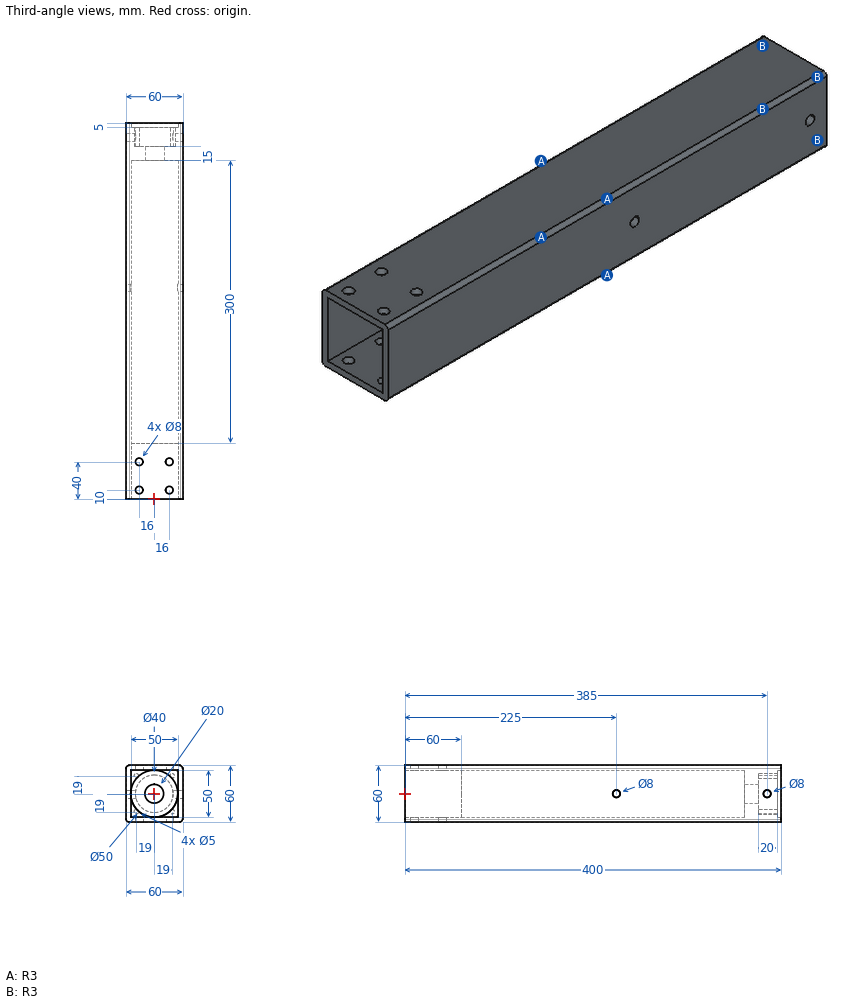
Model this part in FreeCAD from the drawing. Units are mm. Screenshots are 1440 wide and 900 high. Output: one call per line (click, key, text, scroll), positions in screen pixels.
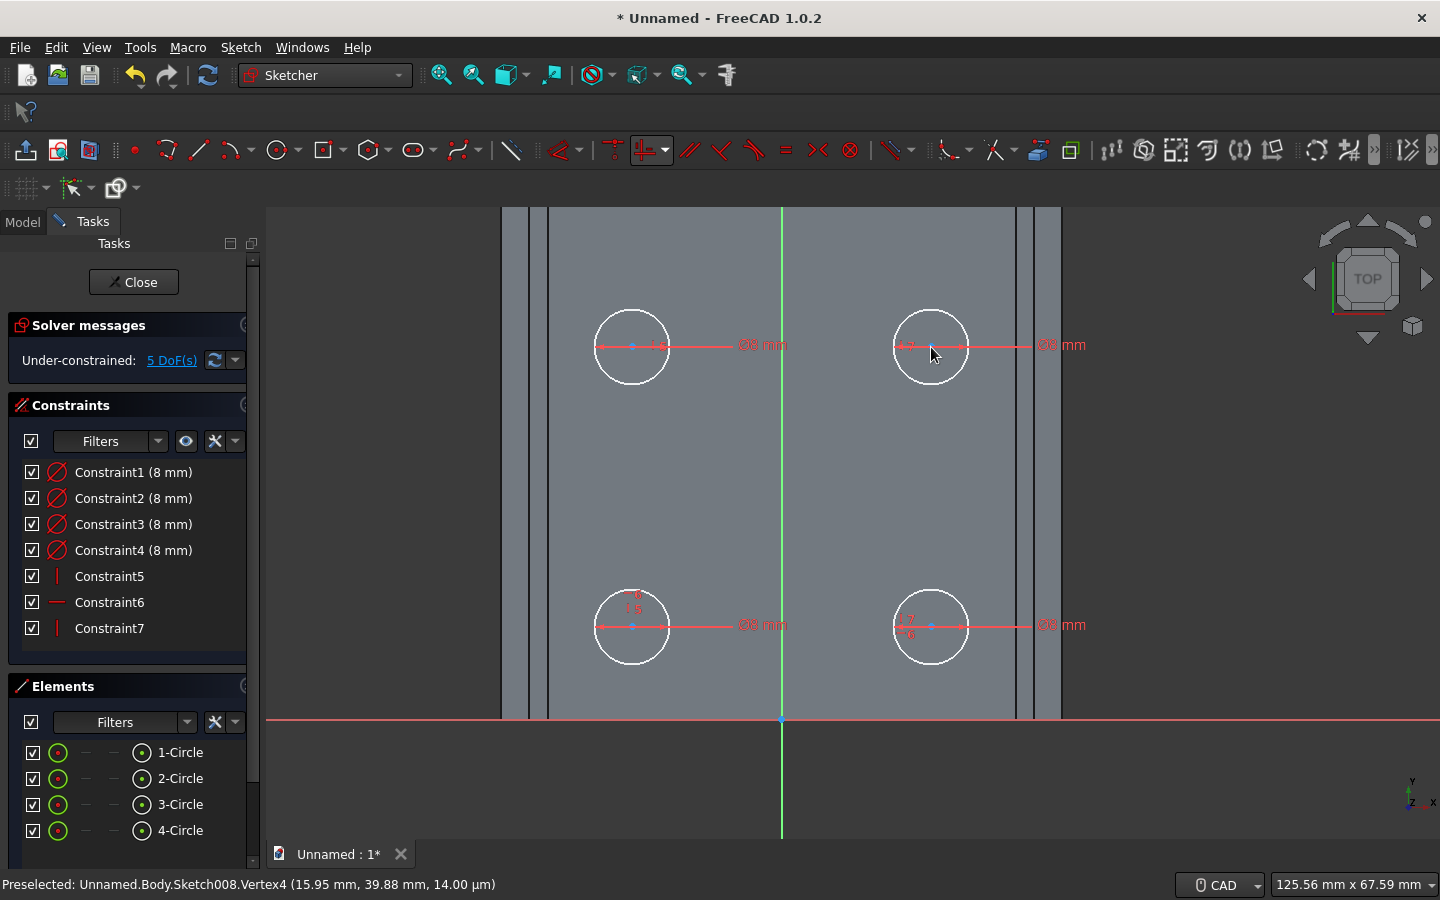
click(632, 347)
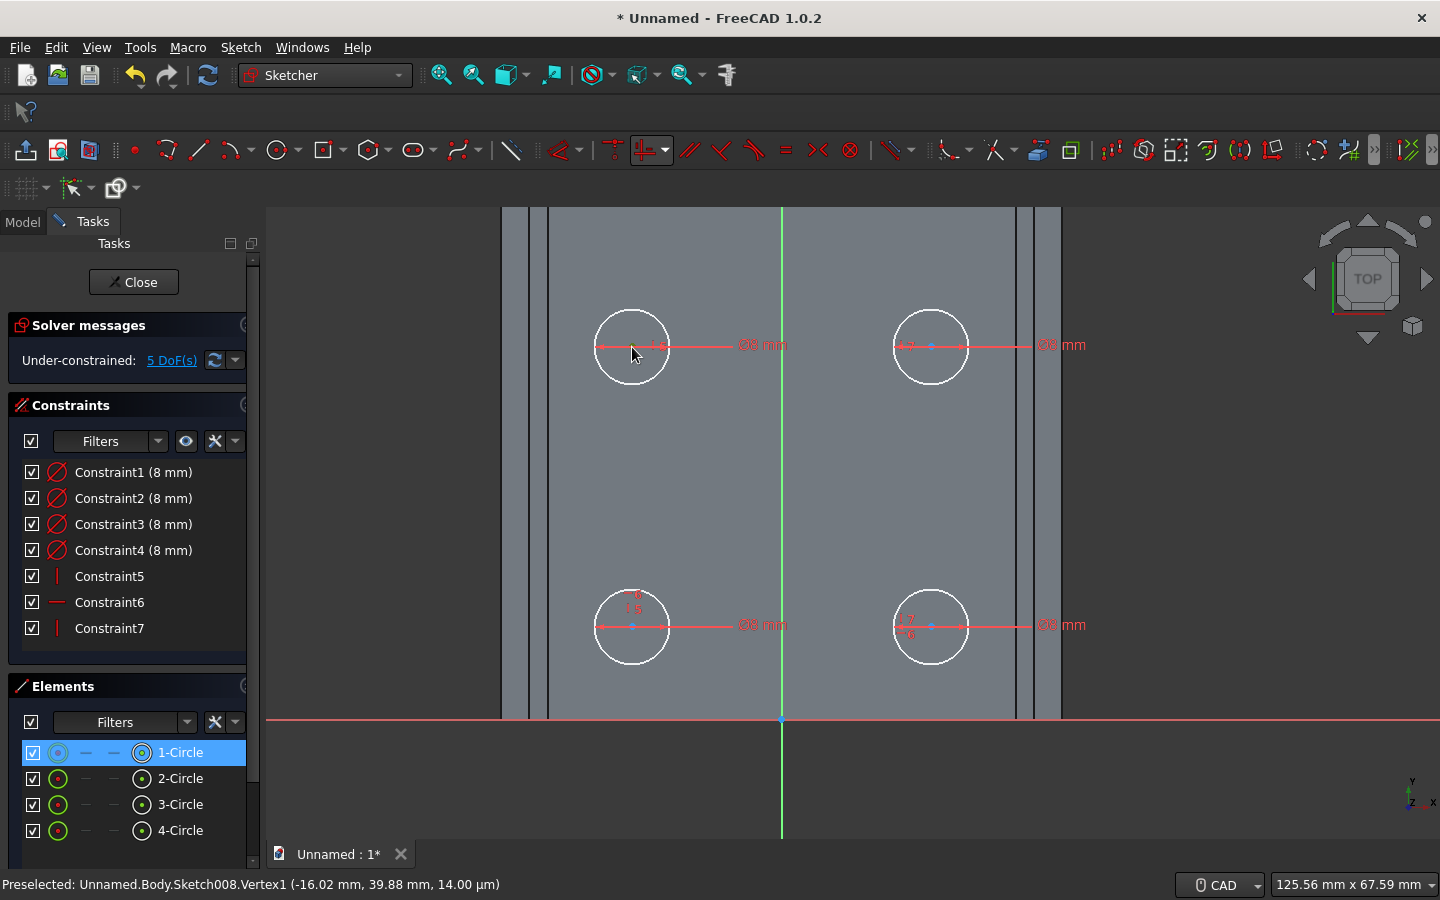
click(931, 347)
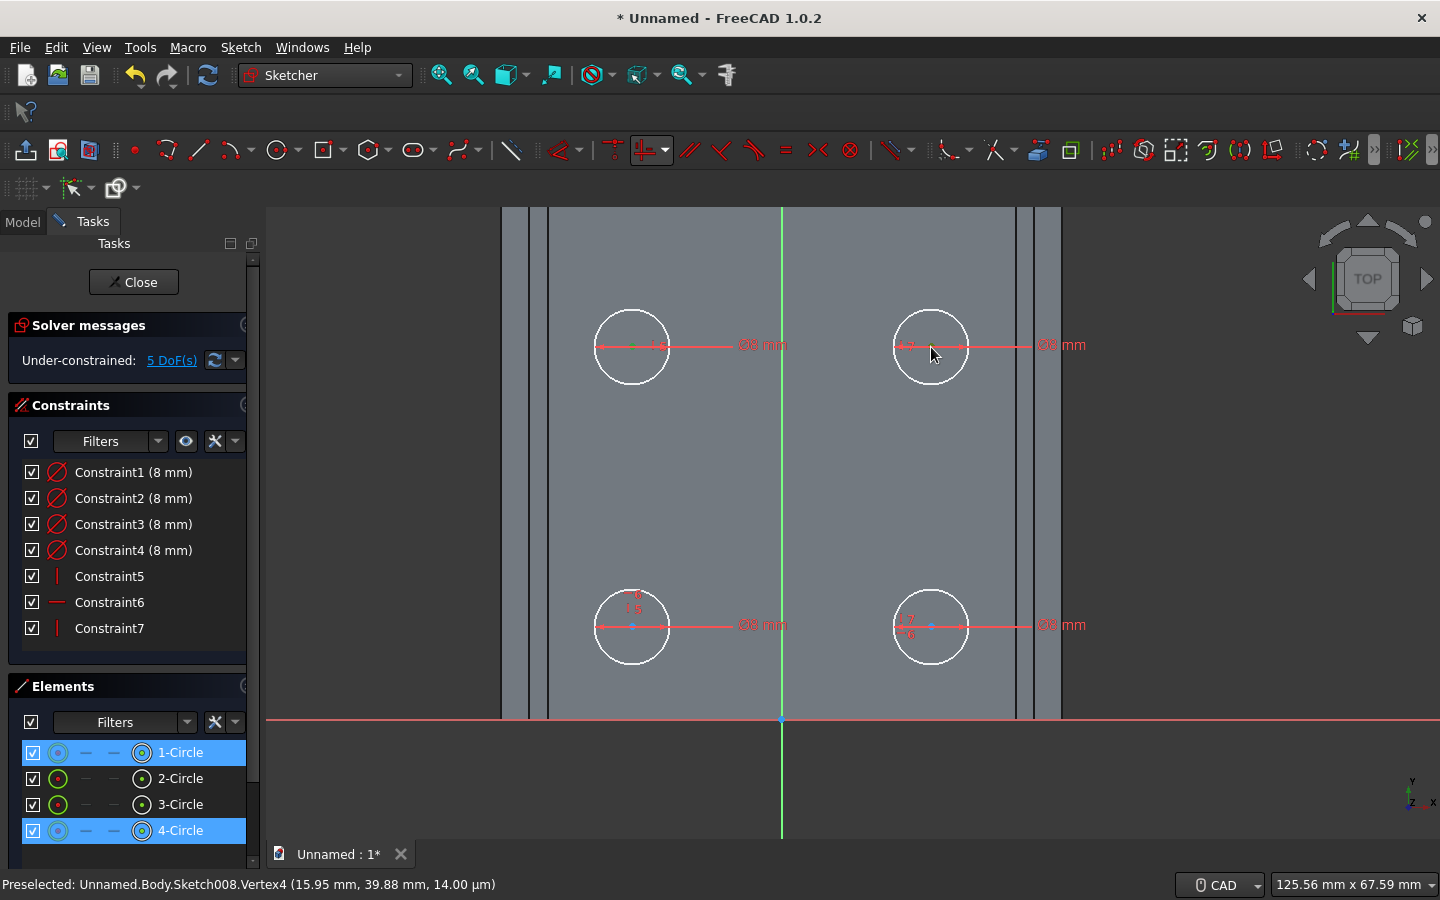
click(668, 150)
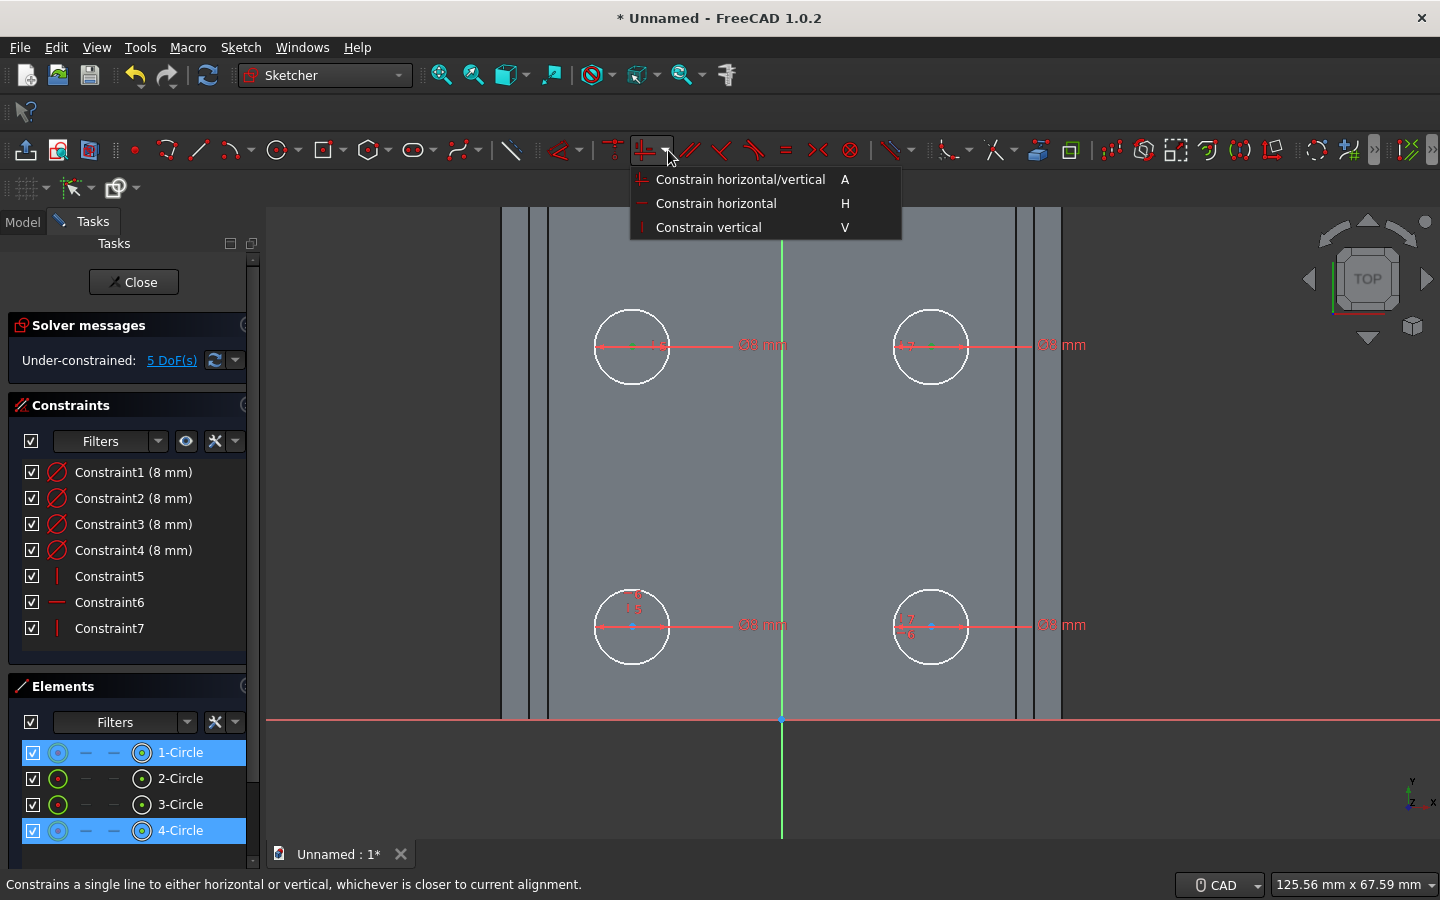
click(766, 203)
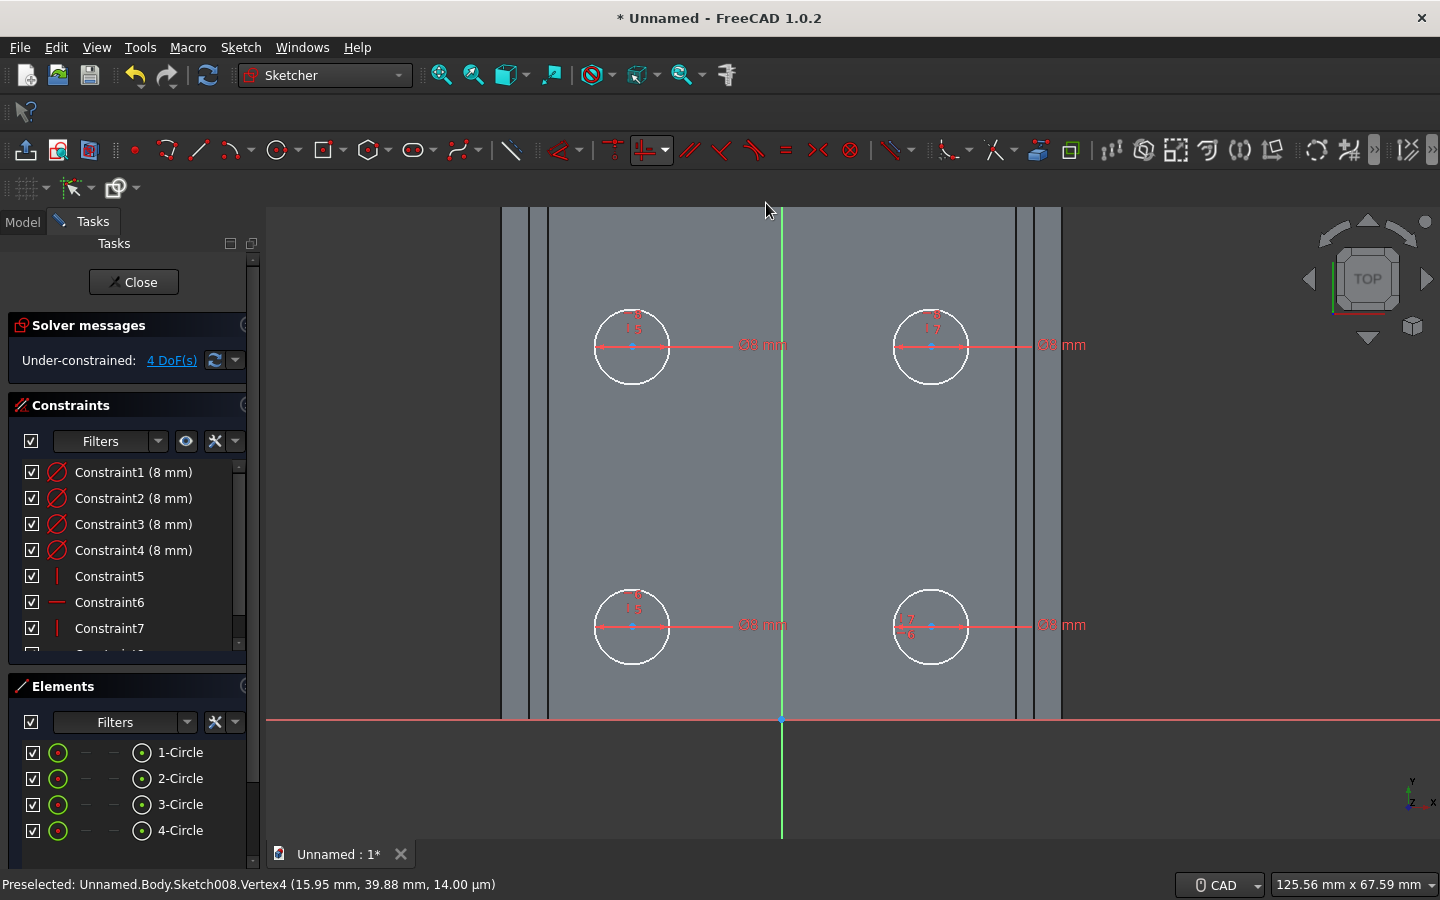
key(d)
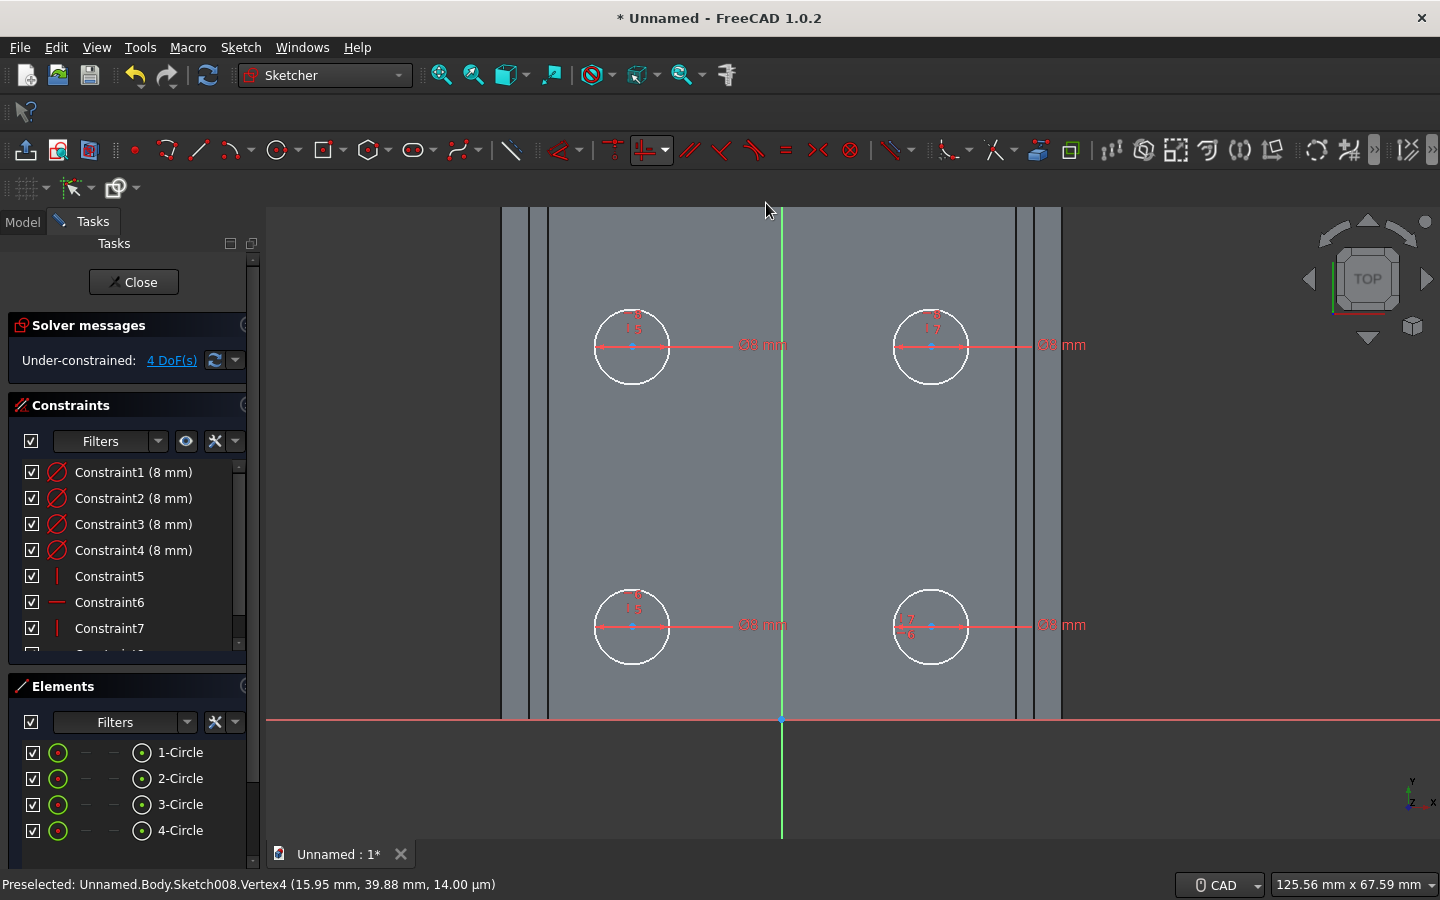
click(632, 347)
click(707, 754)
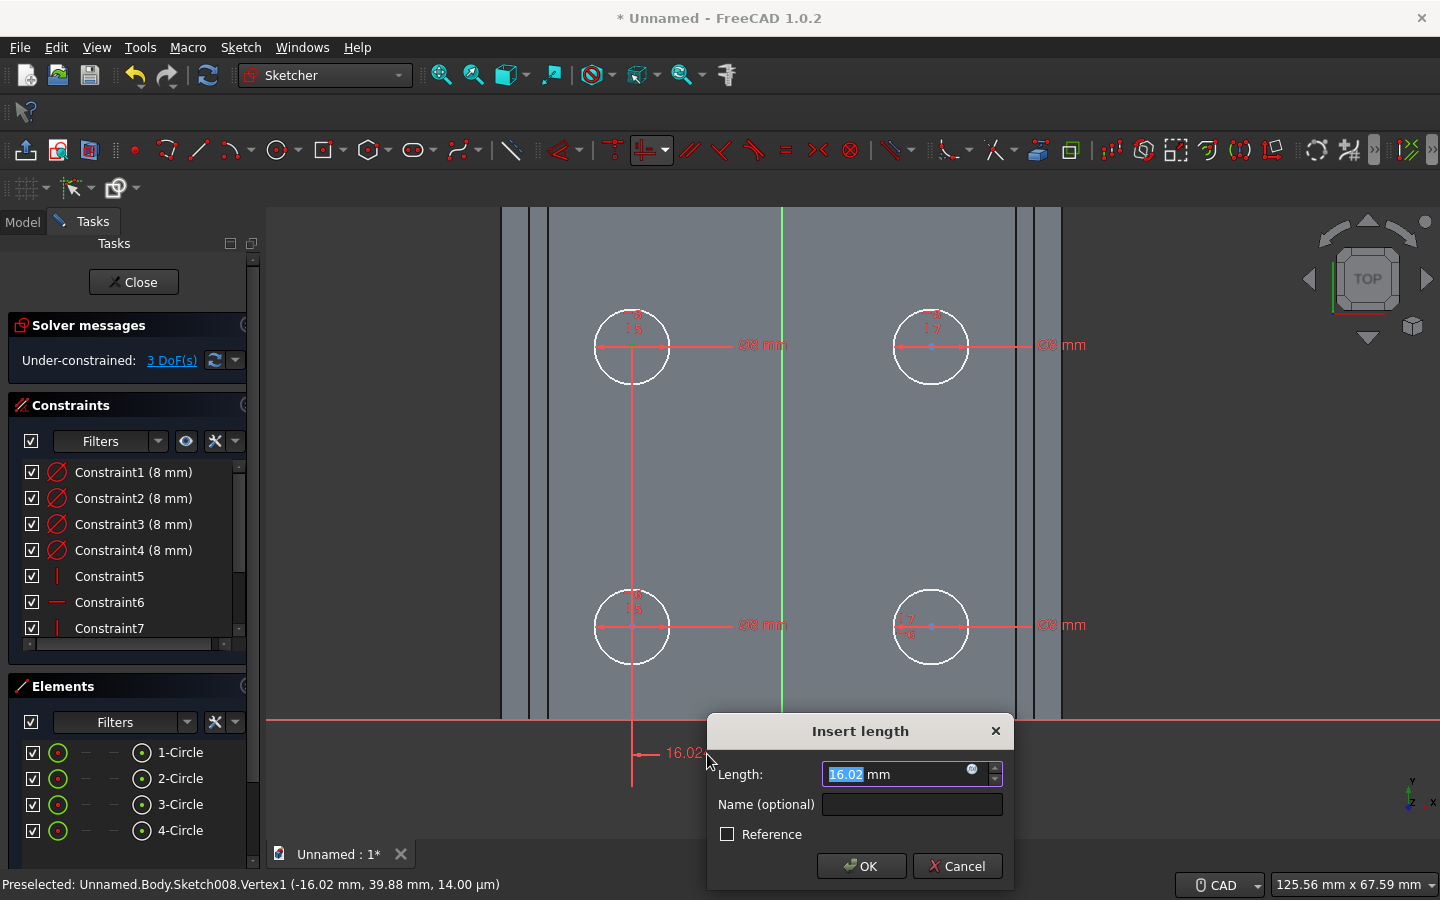
text(16)
key(Return)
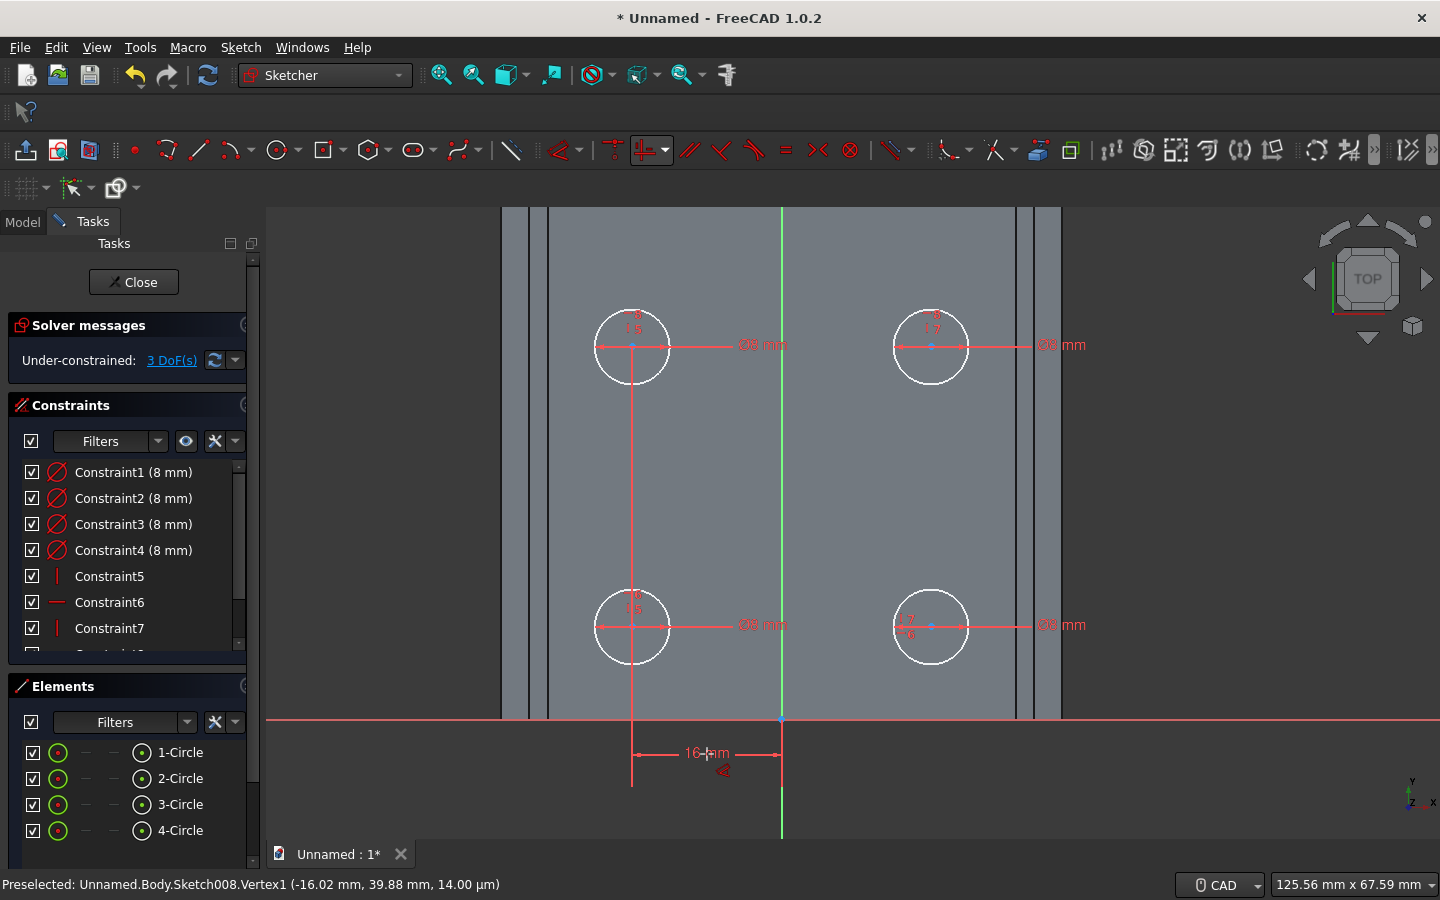
click(632, 347)
click(598, 533)